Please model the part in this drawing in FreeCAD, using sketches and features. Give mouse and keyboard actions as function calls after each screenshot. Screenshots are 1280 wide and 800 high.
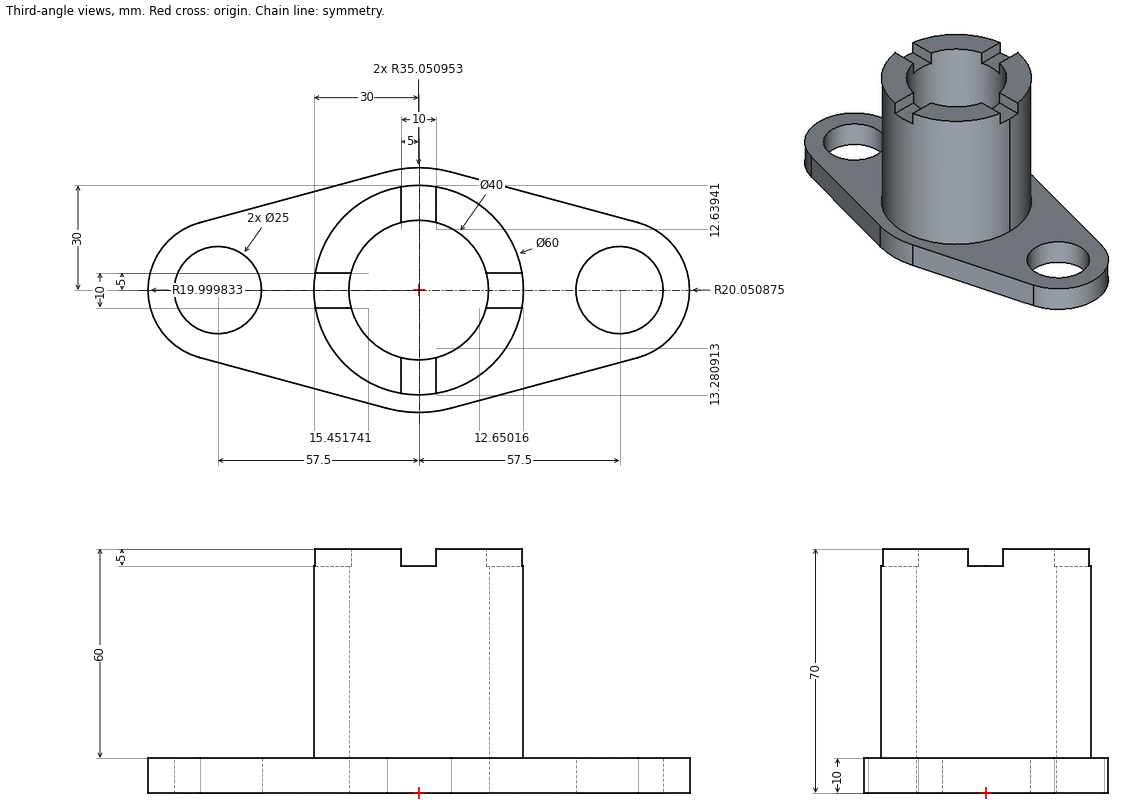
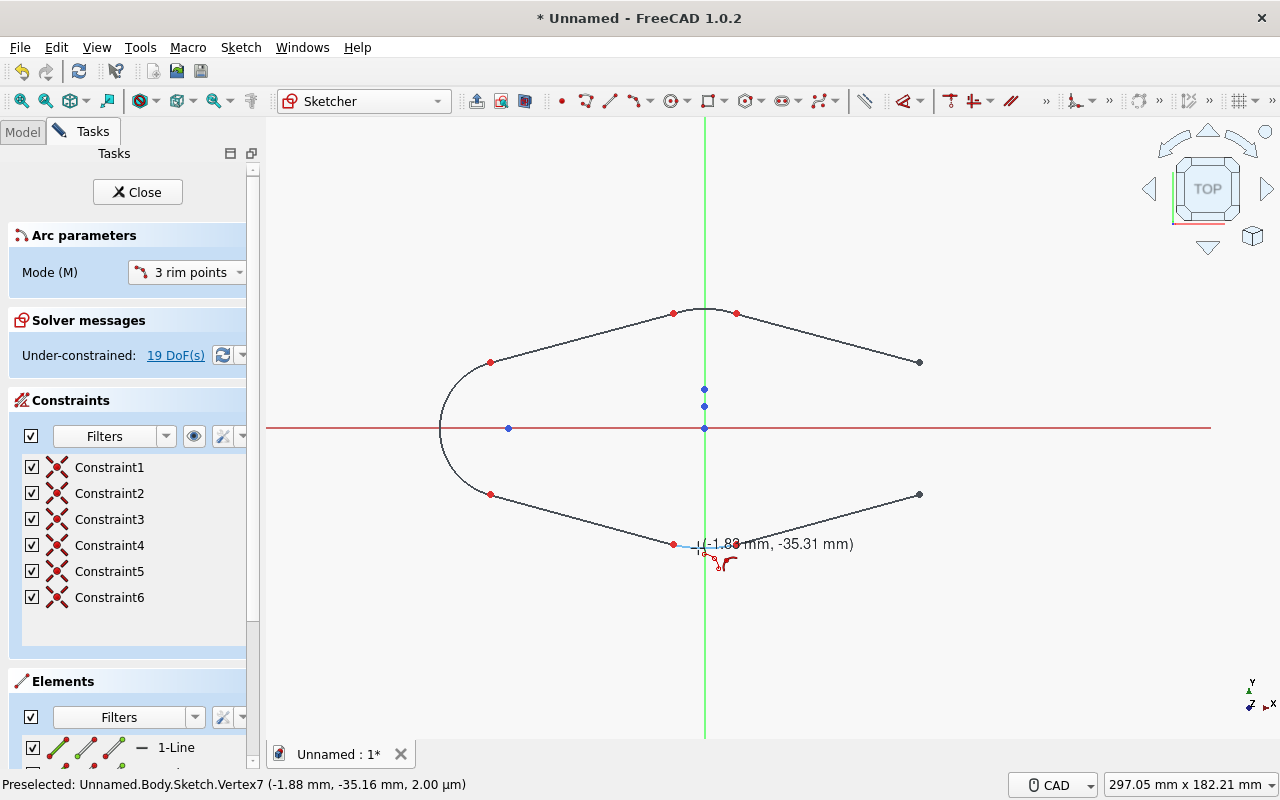
click(919, 495)
click(919, 363)
click(967, 446)
key(Escape)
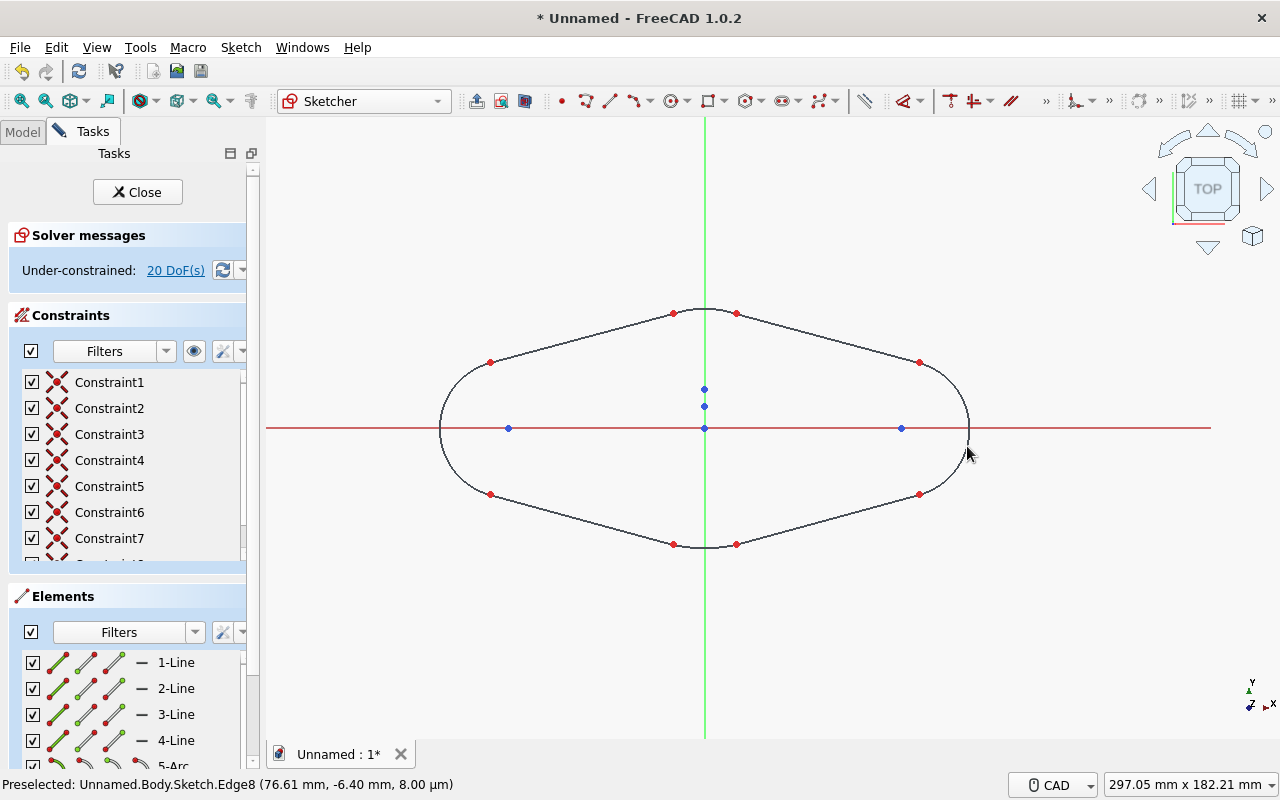
click(864, 348)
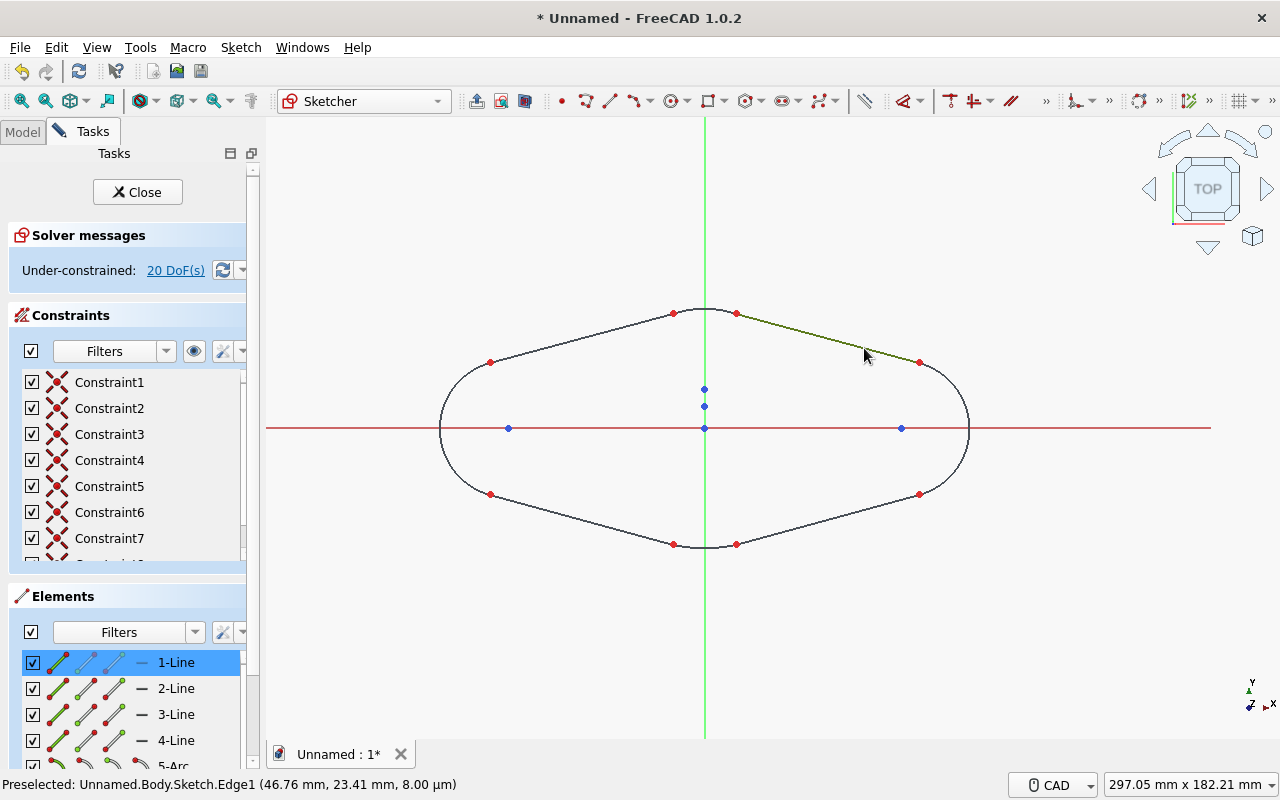
click(717, 310)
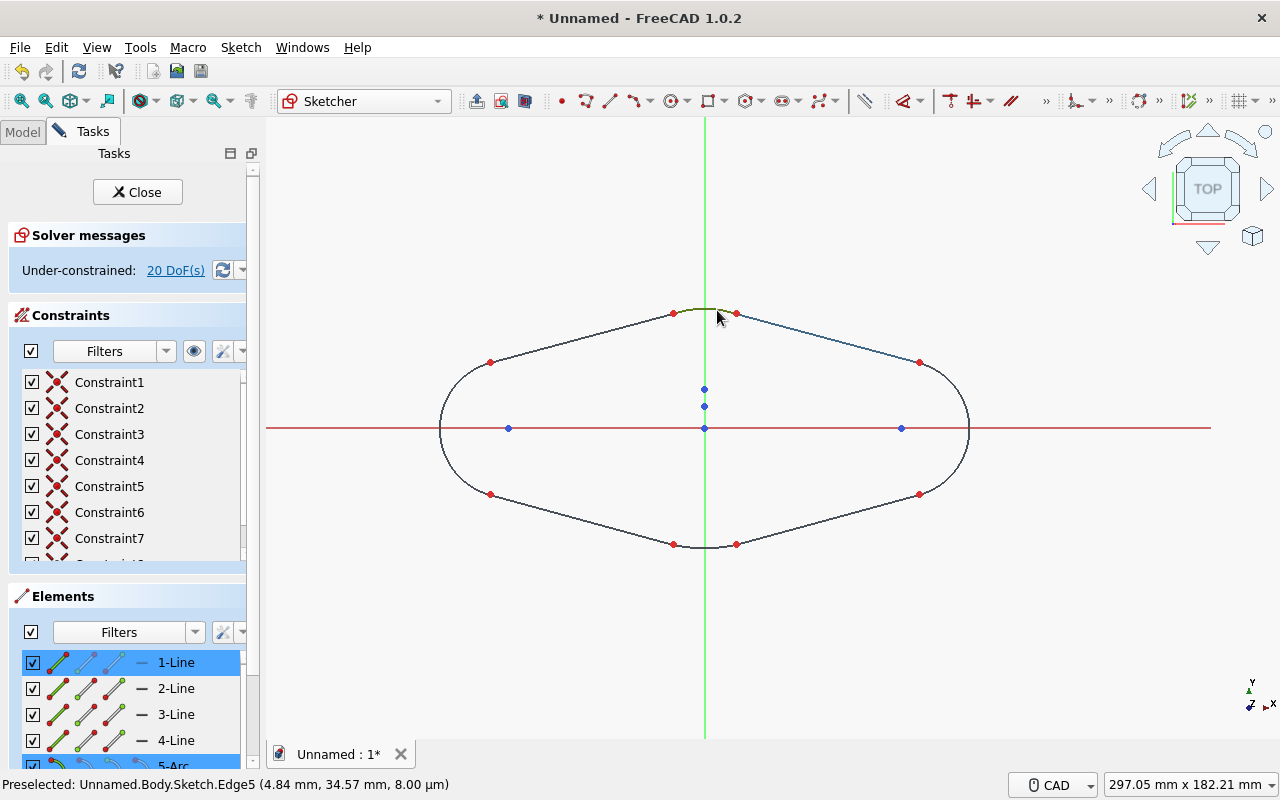
key(t)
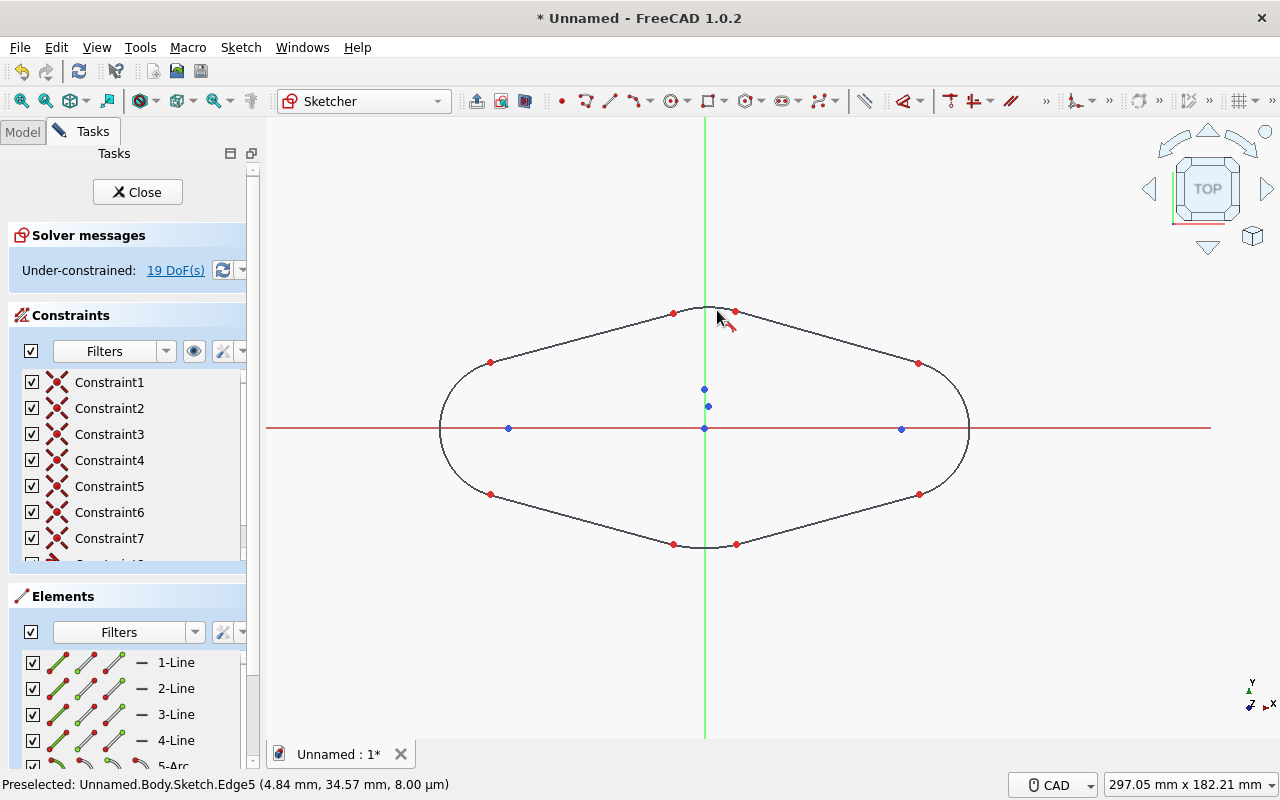
click(864, 347)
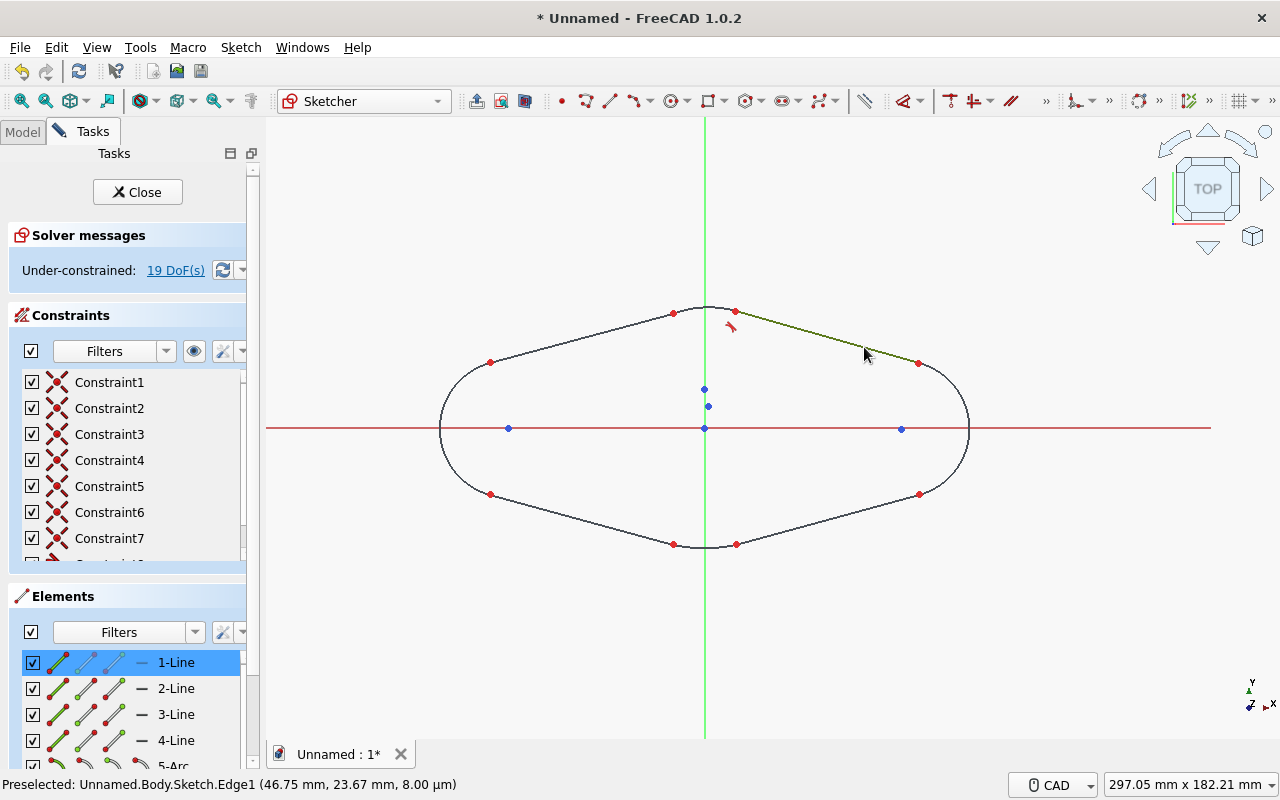
click(960, 463)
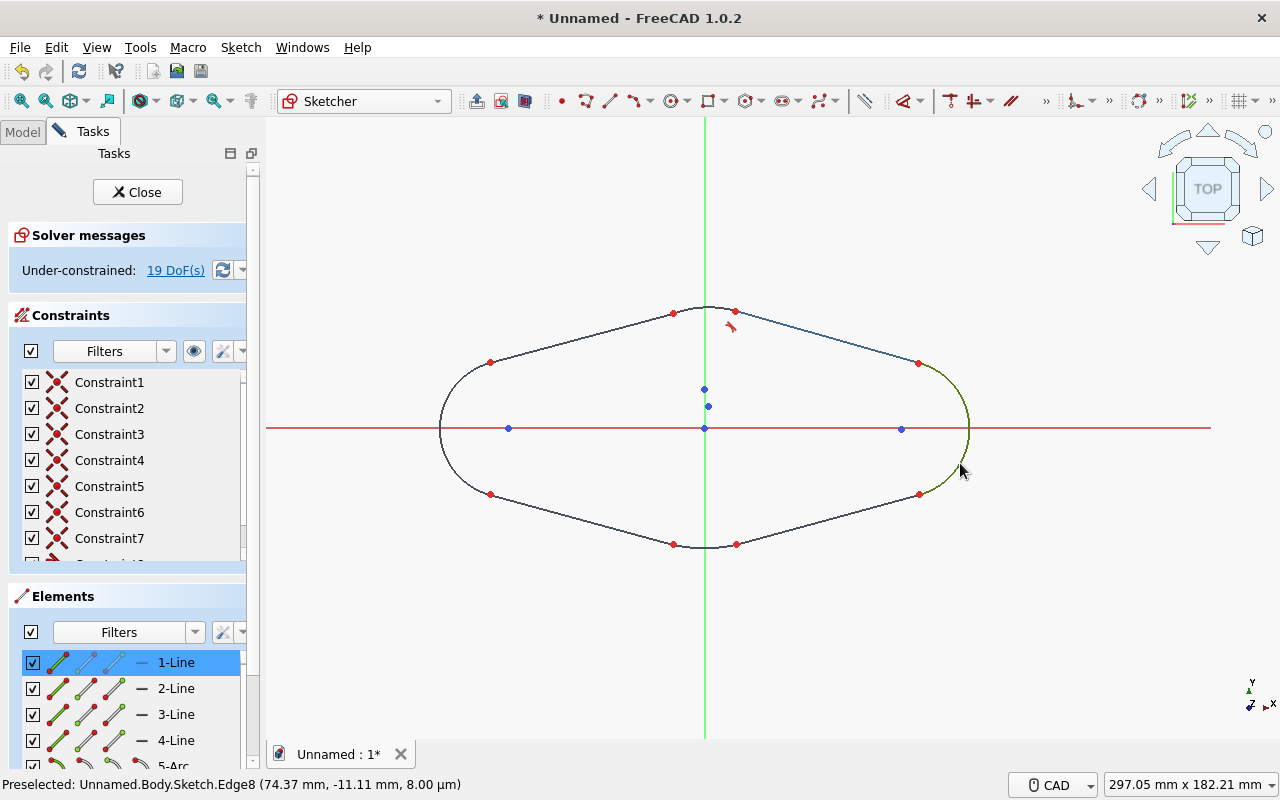
key(t)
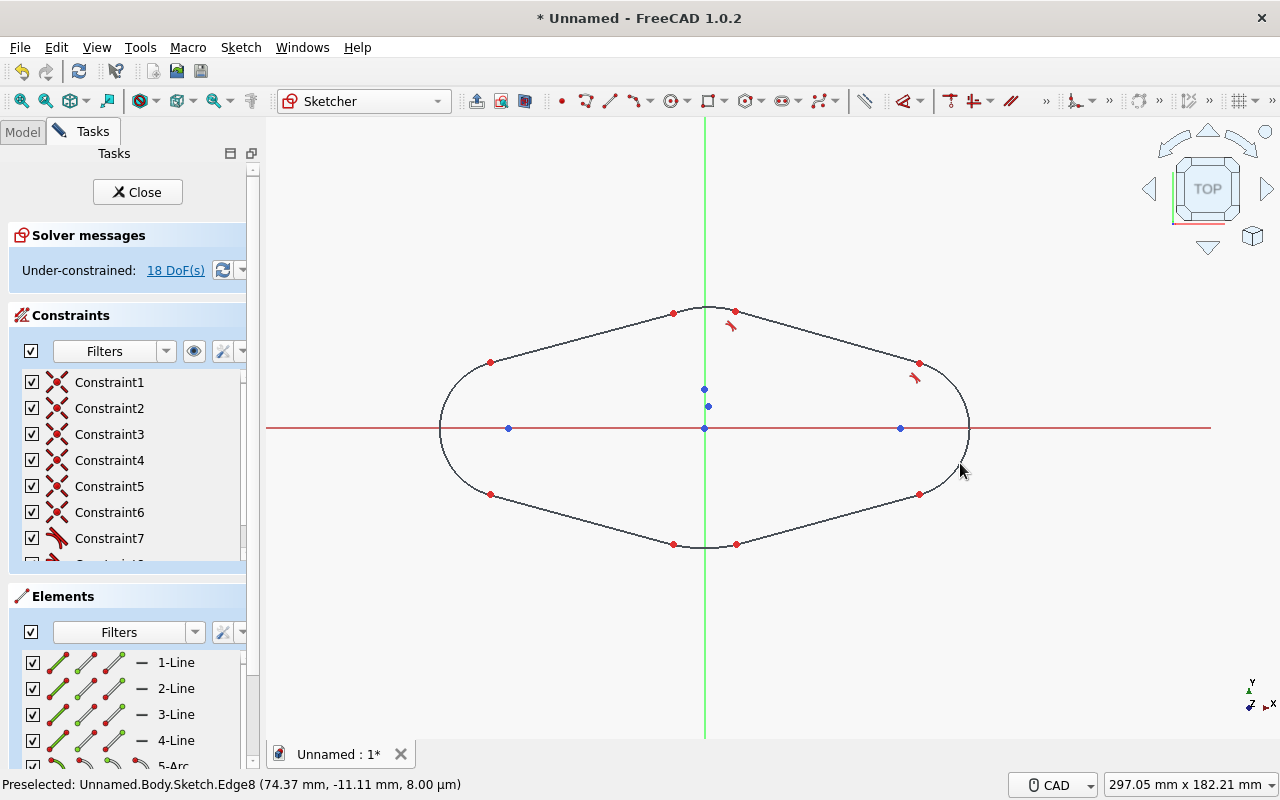
click(618, 329)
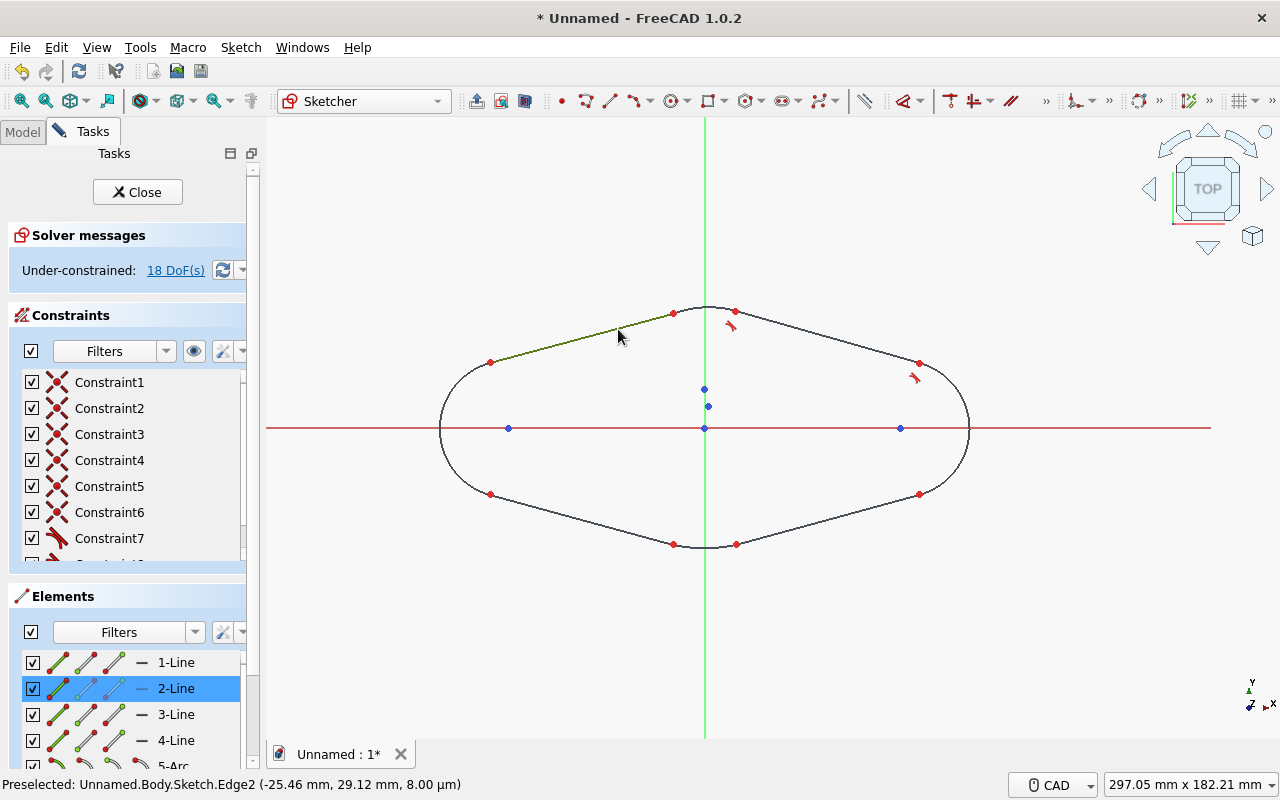
click(717, 308)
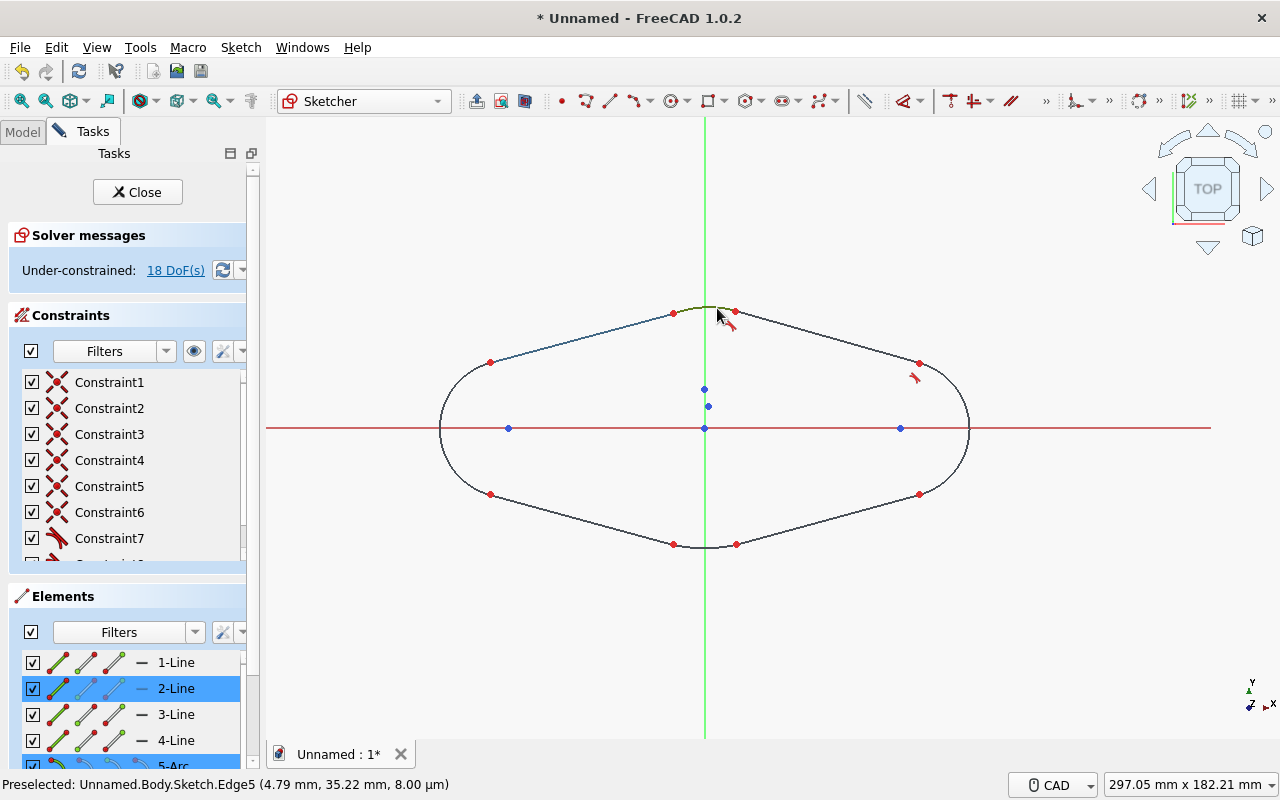
key(t)